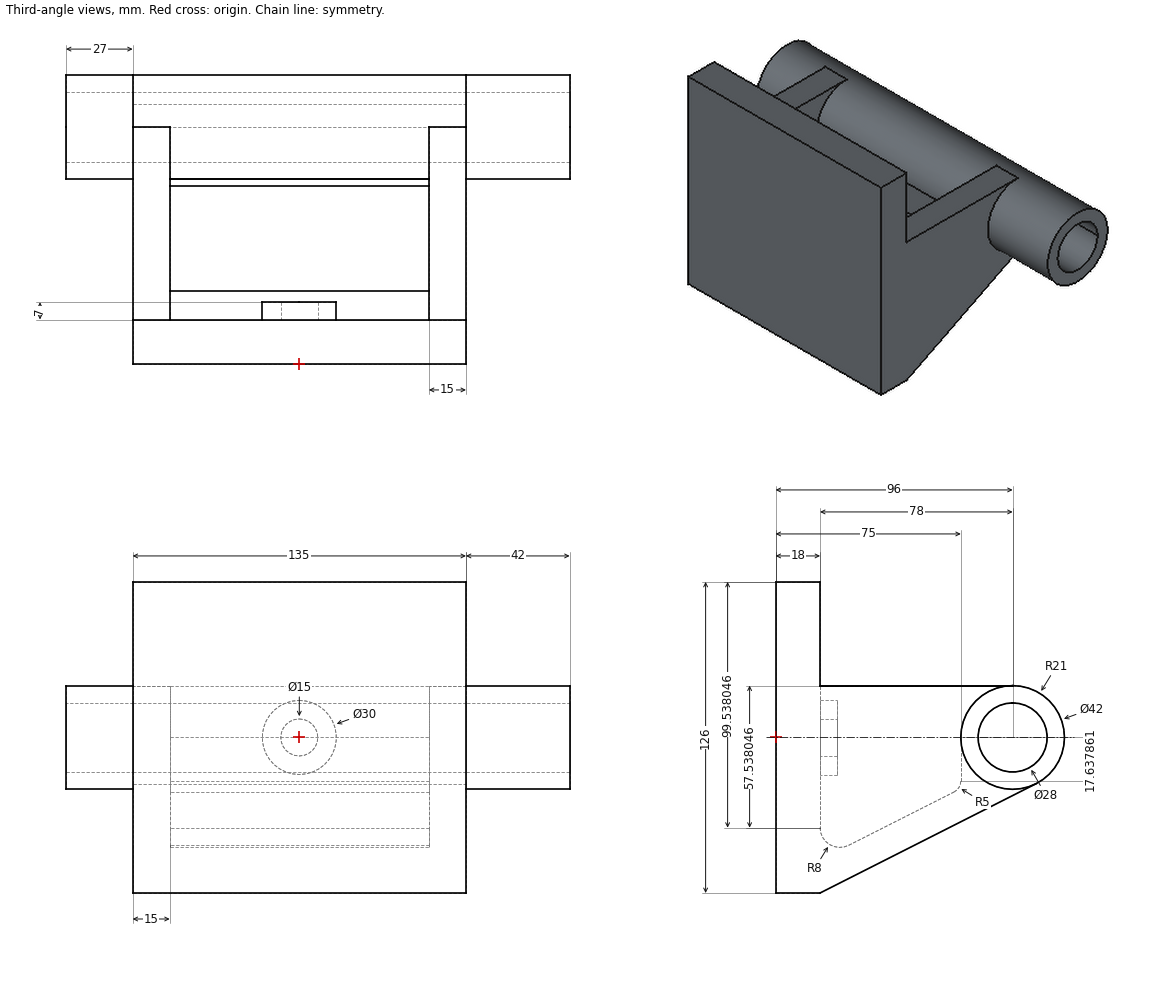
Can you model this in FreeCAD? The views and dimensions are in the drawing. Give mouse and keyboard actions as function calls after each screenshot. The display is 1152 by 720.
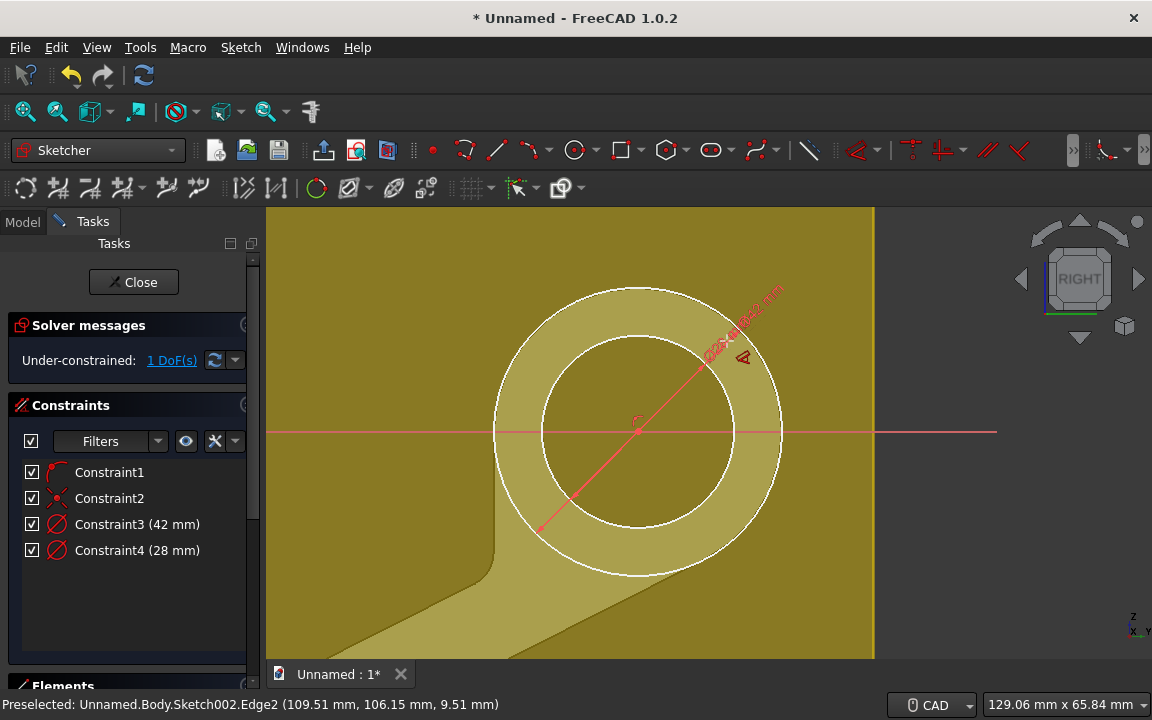
click(638, 432)
click(466, 466)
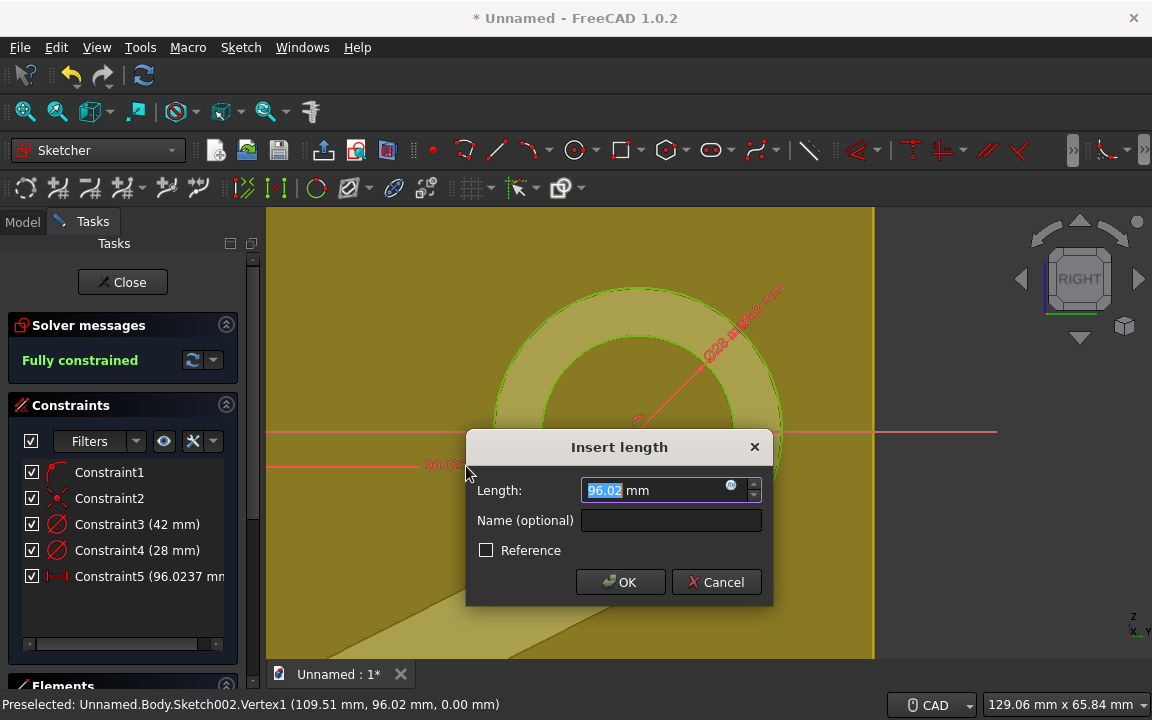
text(96)
key(Return)
key(Escape)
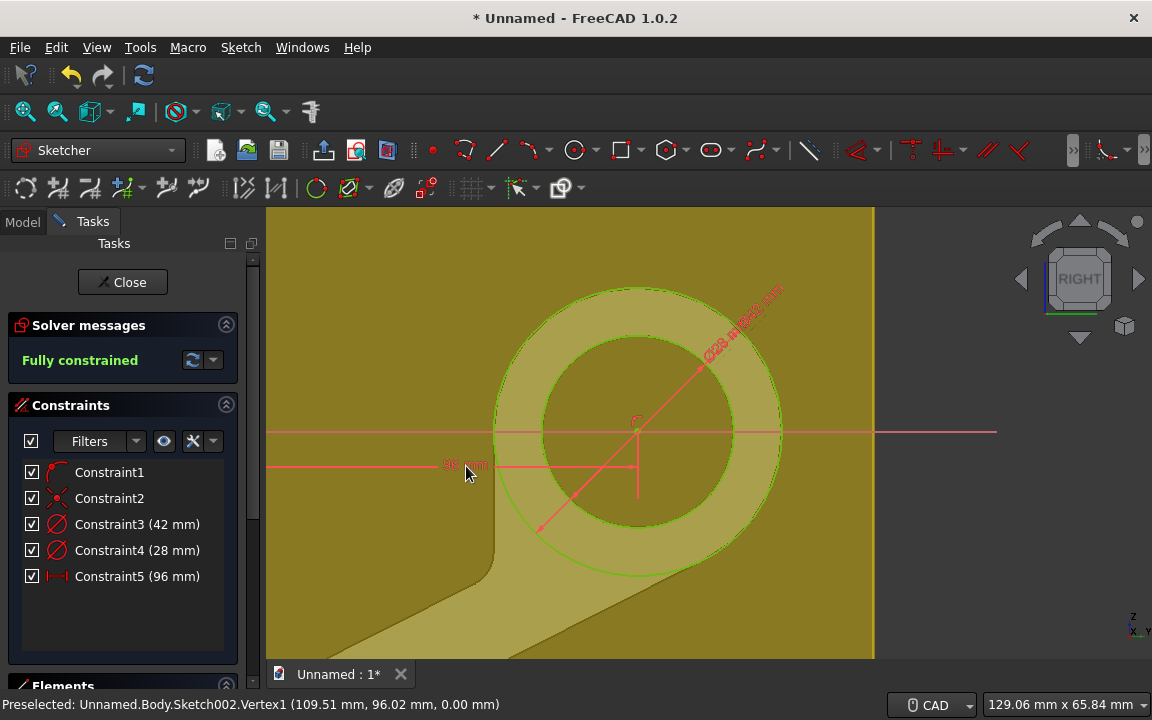
click(123, 282)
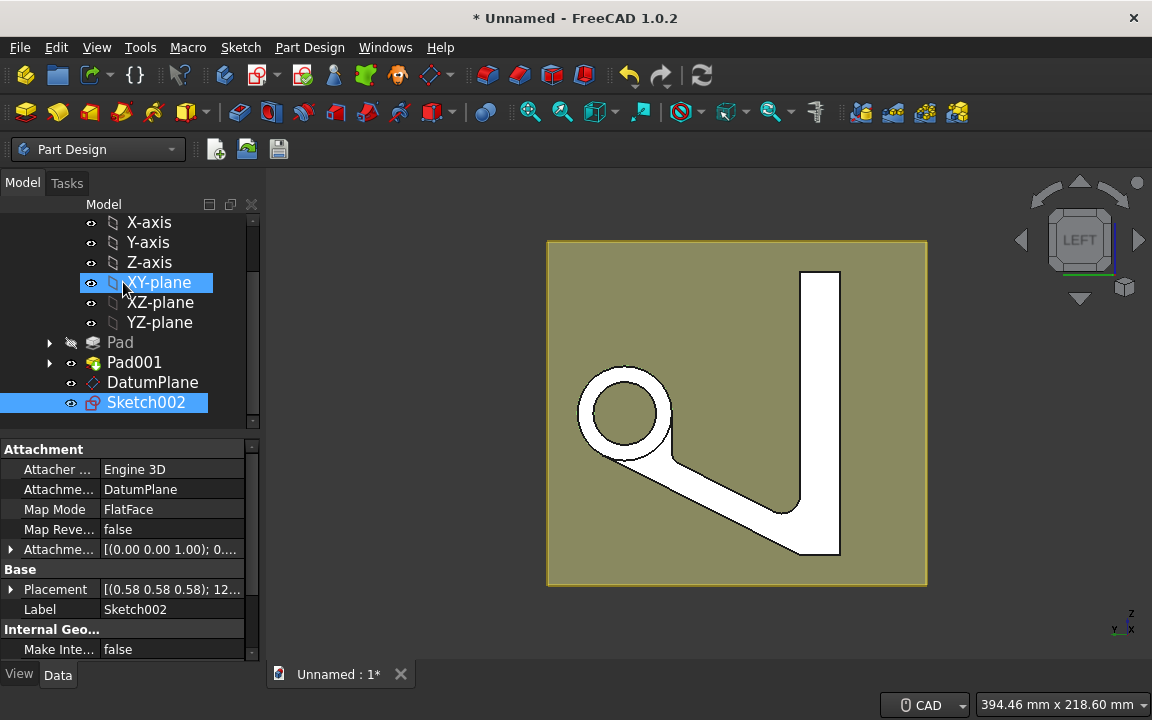
click(26, 112)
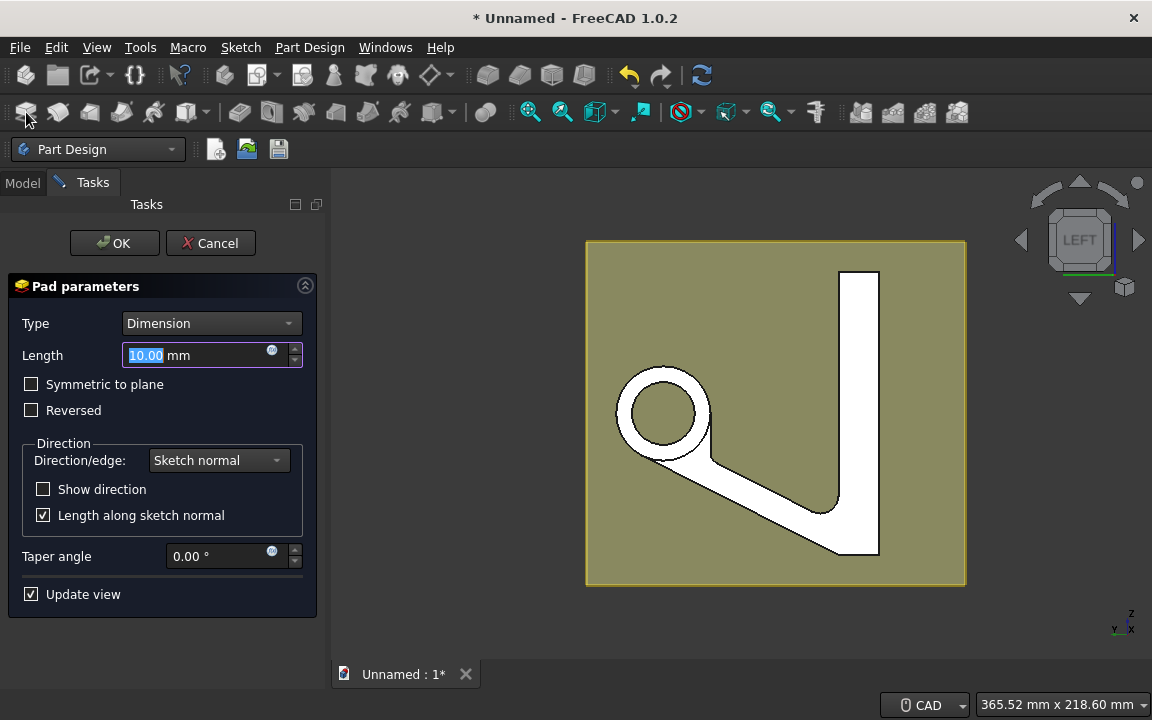
text(42)
key(Tab)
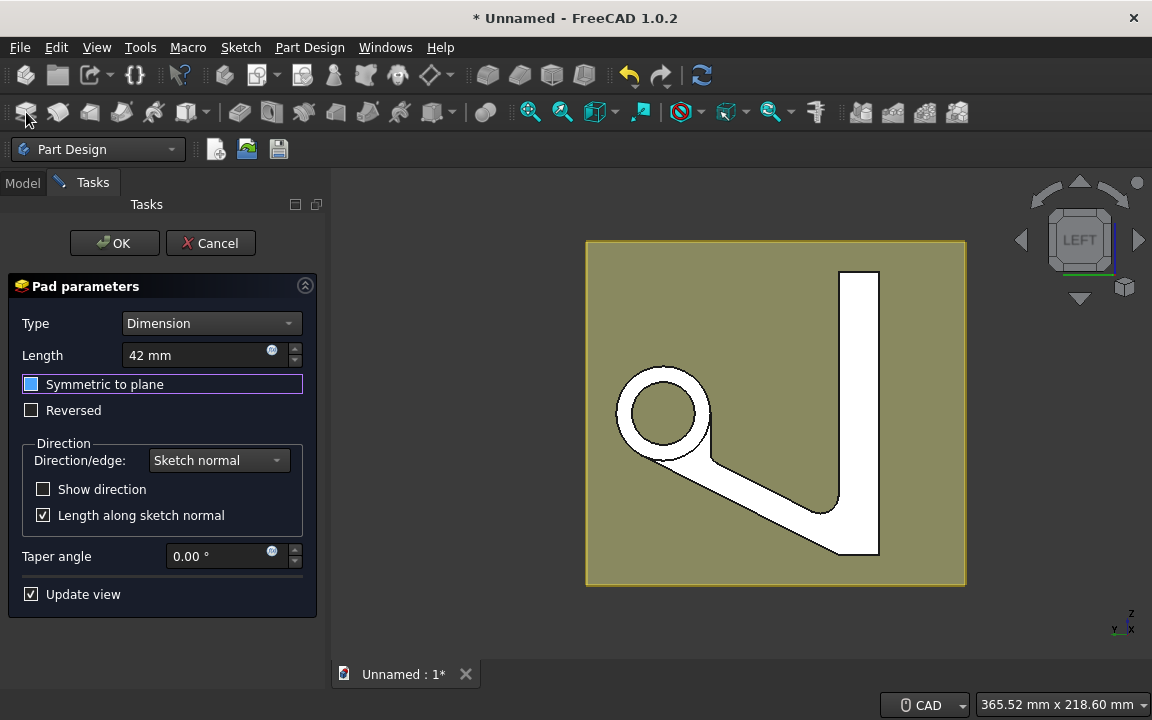
click(30, 410)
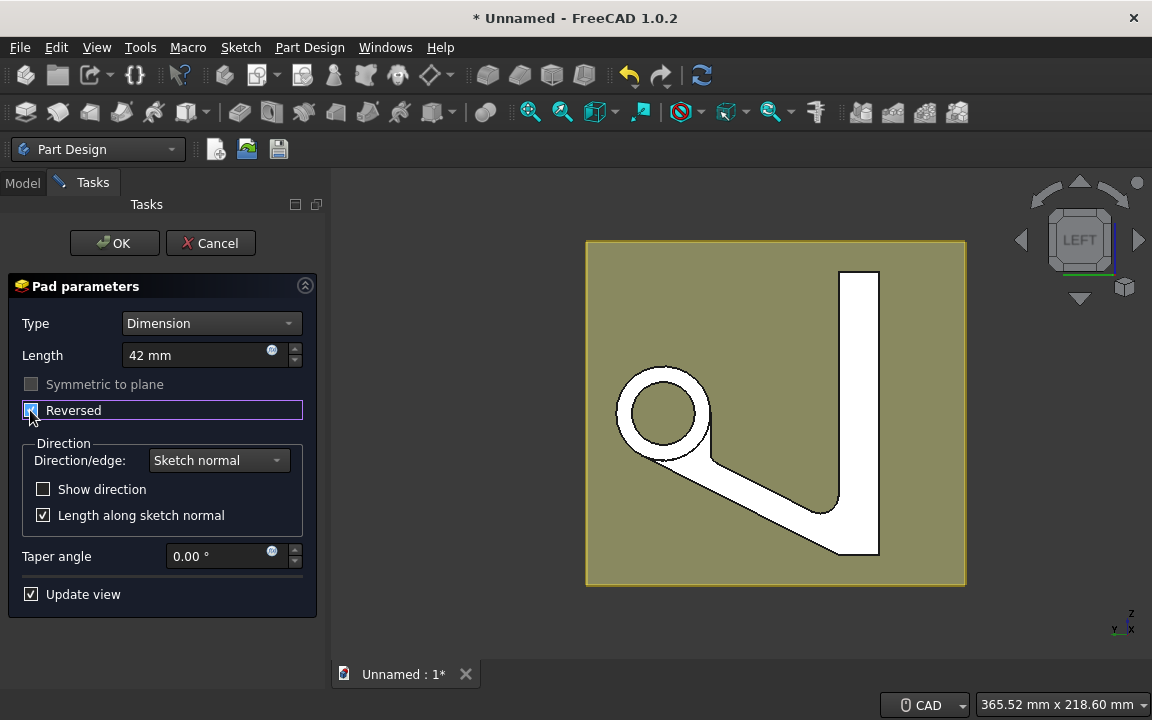
click(115, 243)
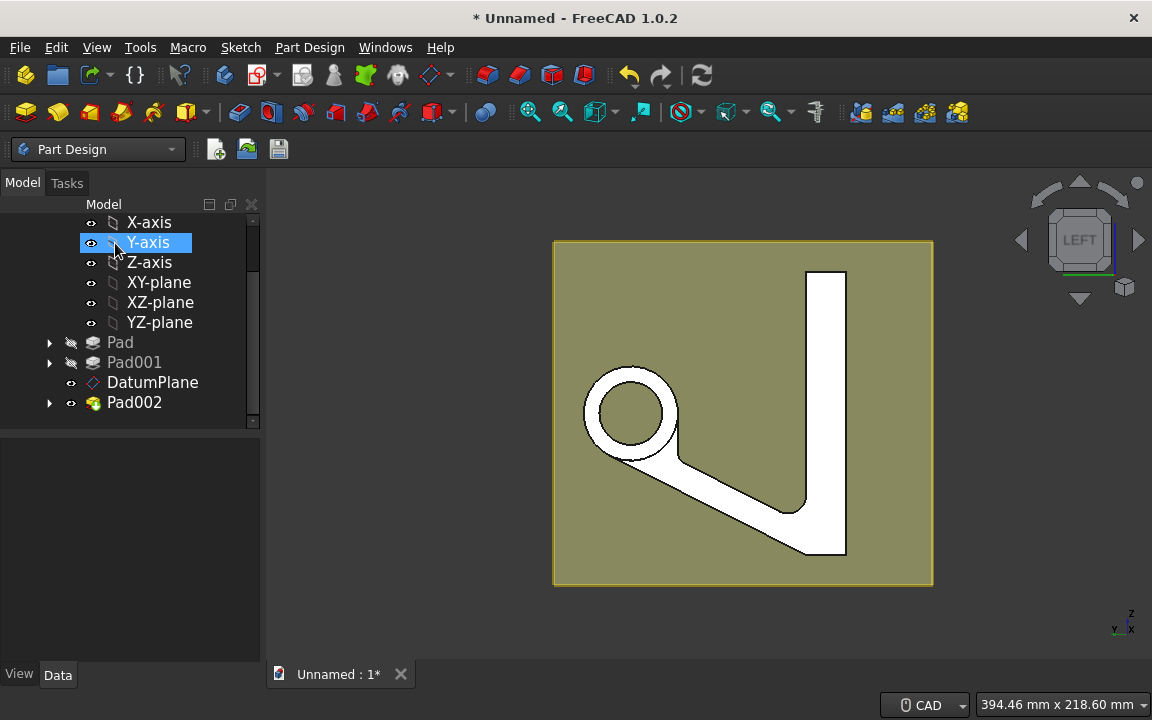
click(116, 383)
key(space)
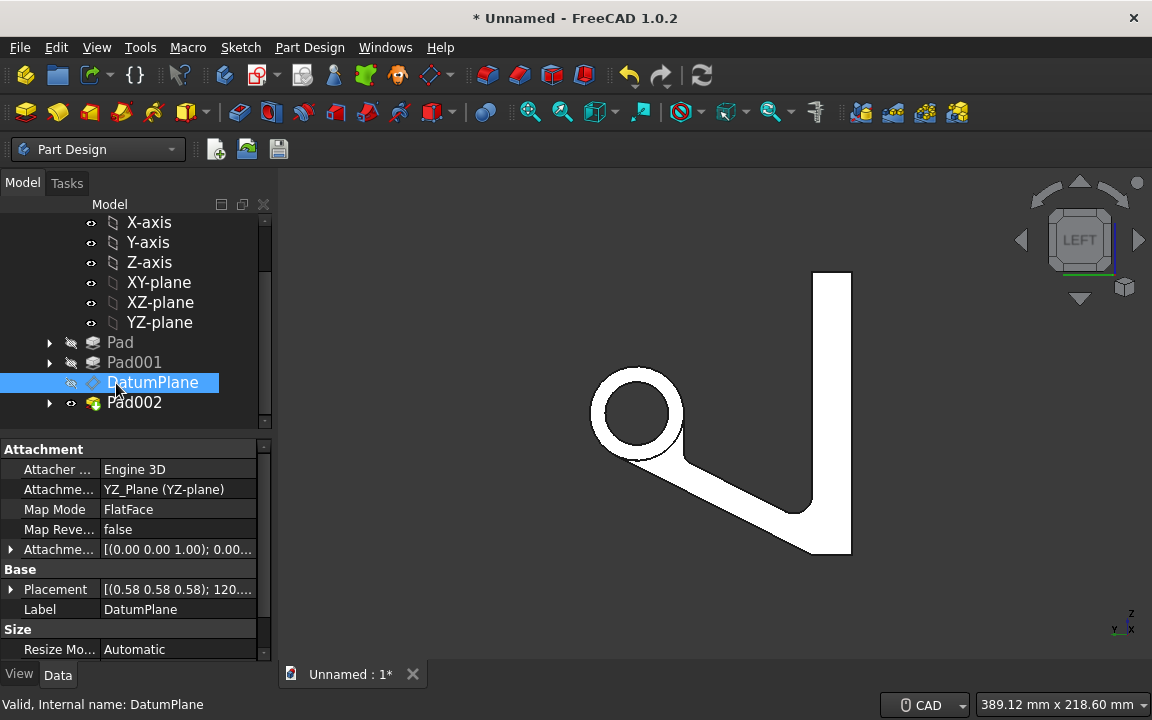
key(0)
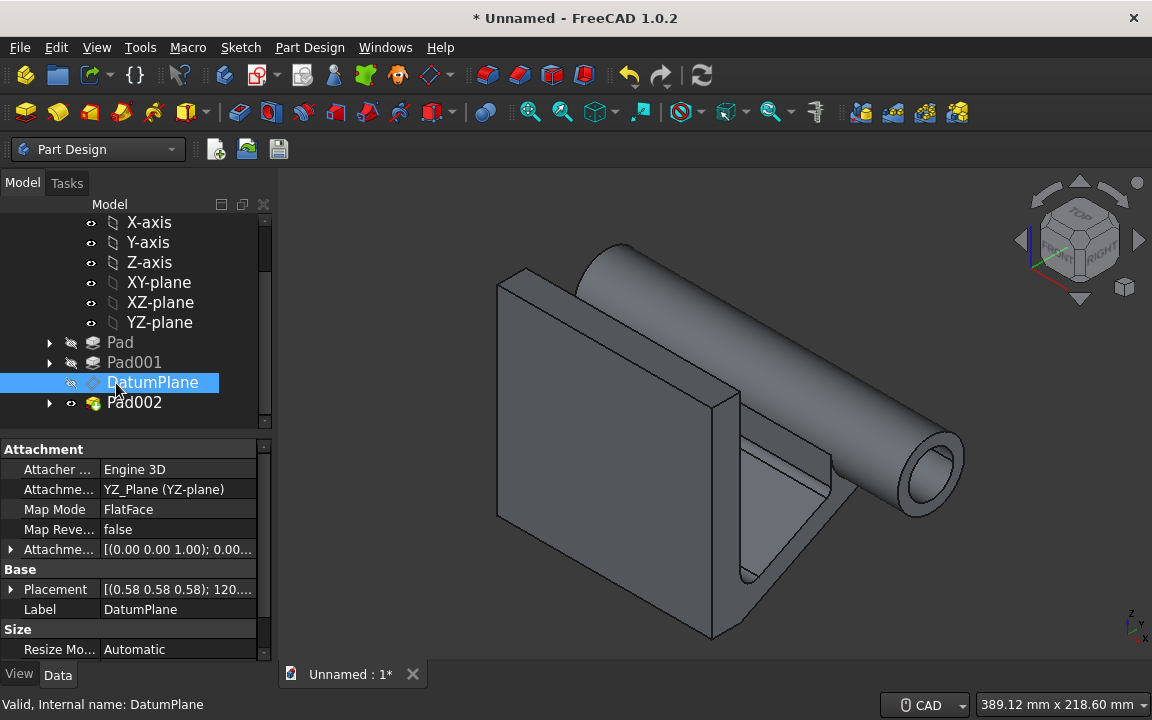
click(532, 112)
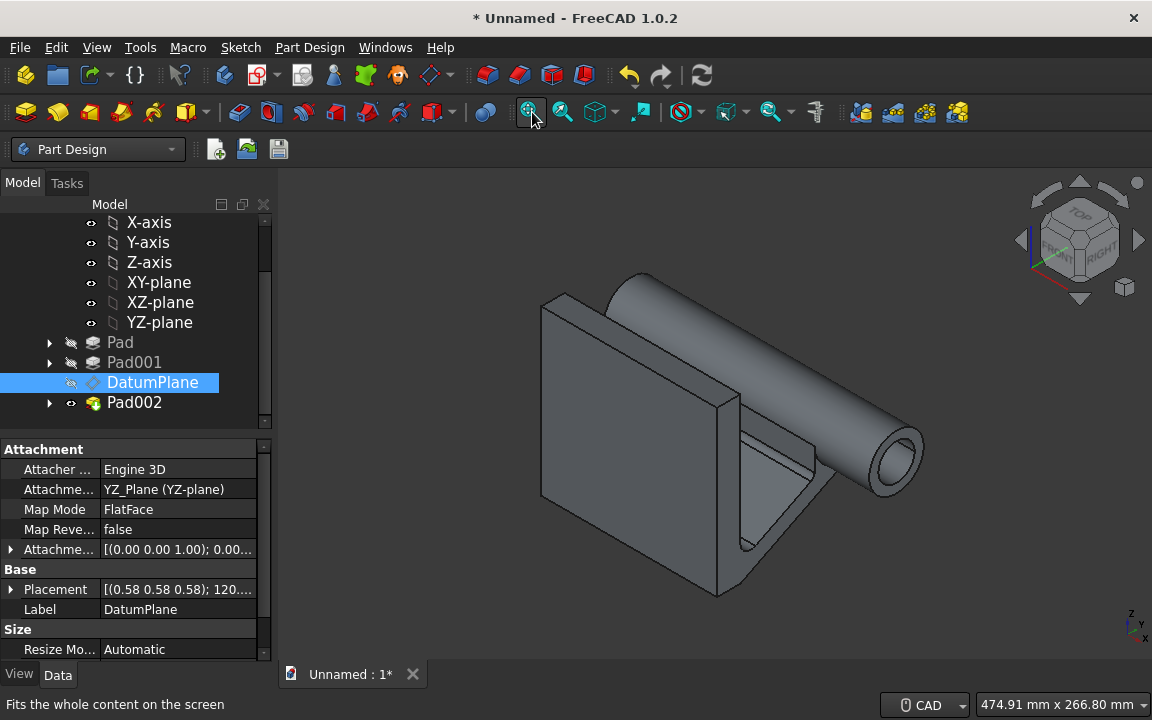
click(727, 577)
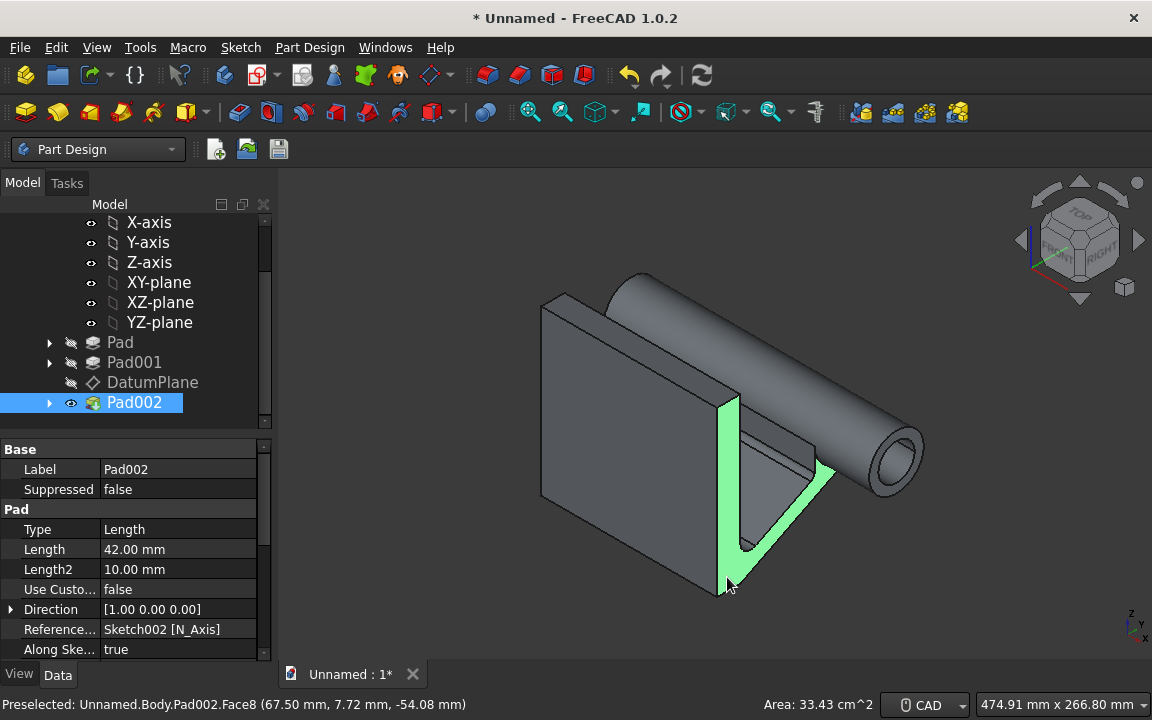
click(258, 76)